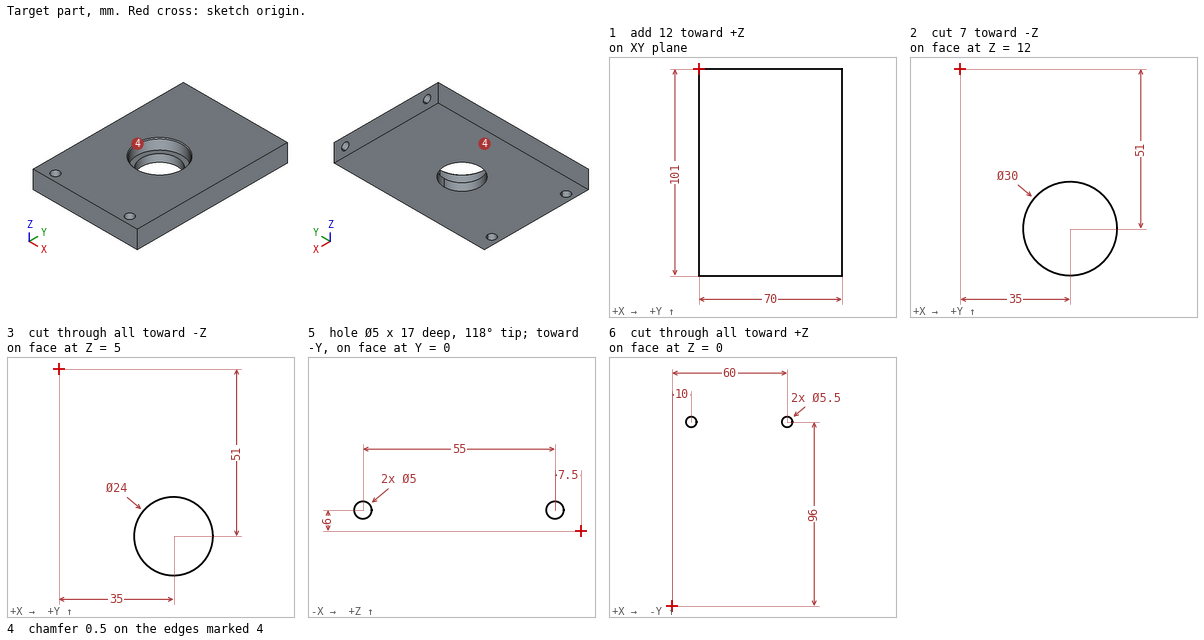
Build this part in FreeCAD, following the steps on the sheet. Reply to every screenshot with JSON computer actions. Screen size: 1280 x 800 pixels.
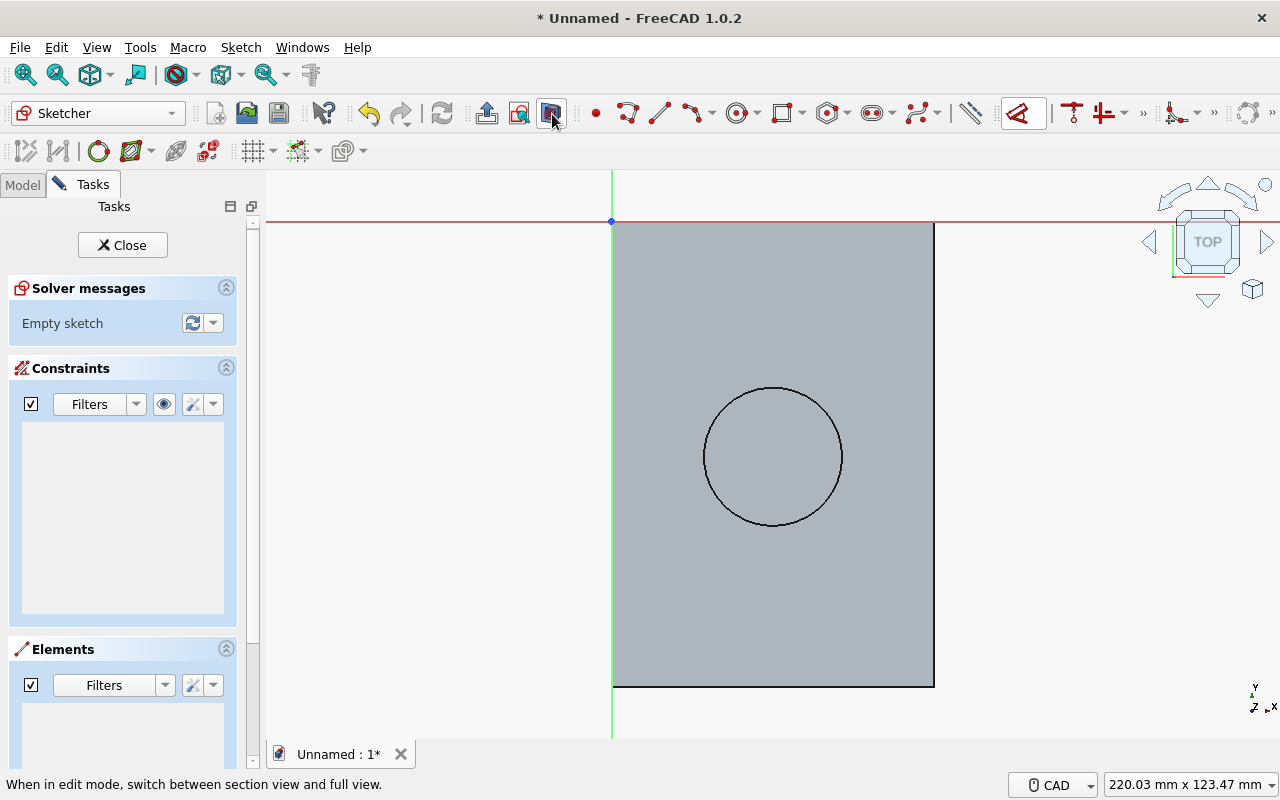
{"action": "scroll", "coordinate": [803, 458], "scroll_direction": "up", "scroll_amount": 6}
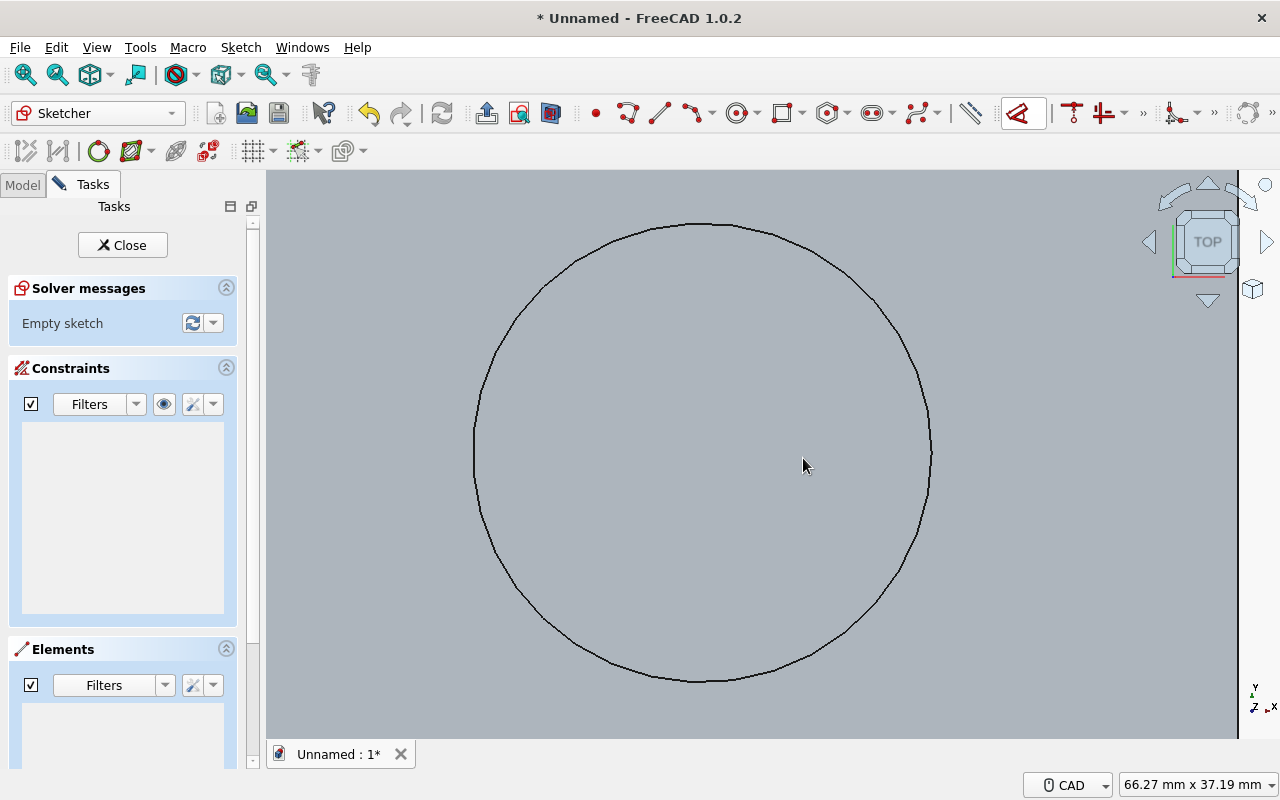
{"action": "left_click", "coordinate": [738, 114]}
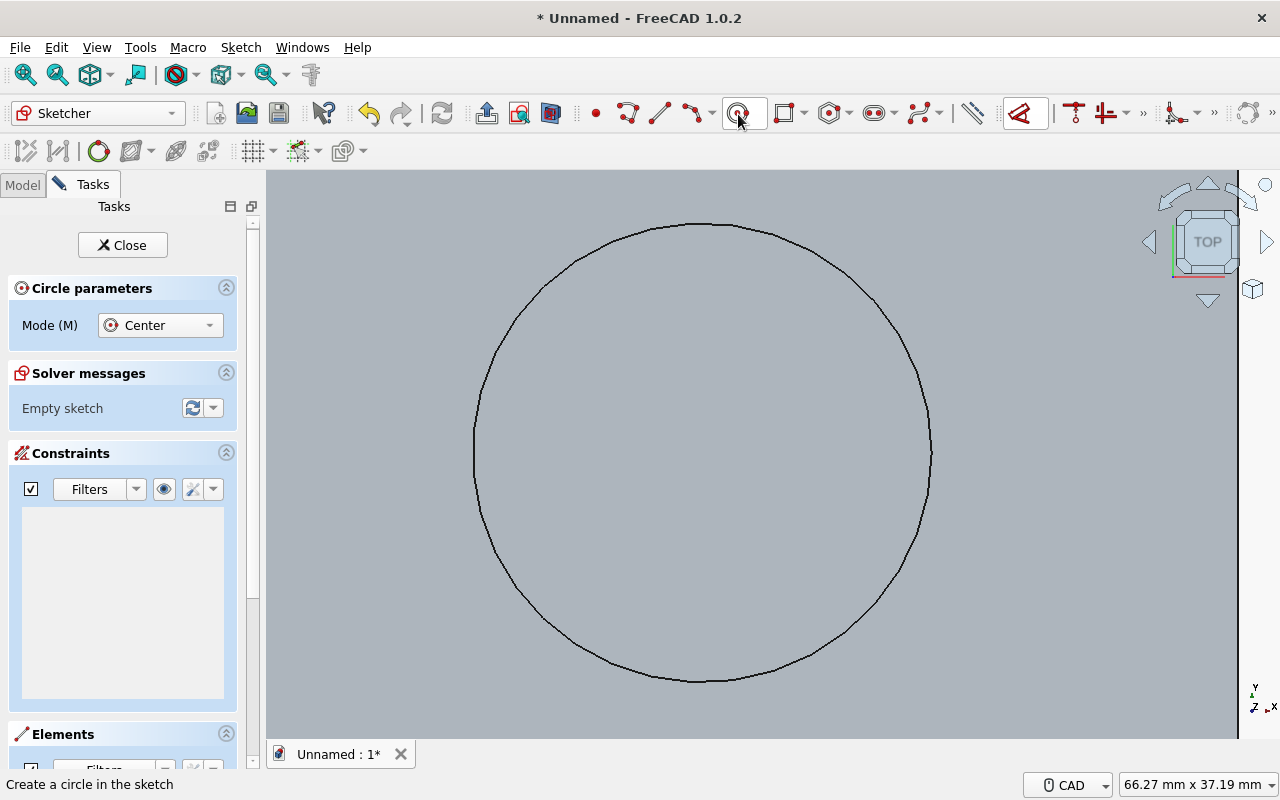
{"action": "left_click", "coordinate": [702, 453]}
{"action": "left_click", "coordinate": [832, 323]}
{"action": "key", "text": "Escape"}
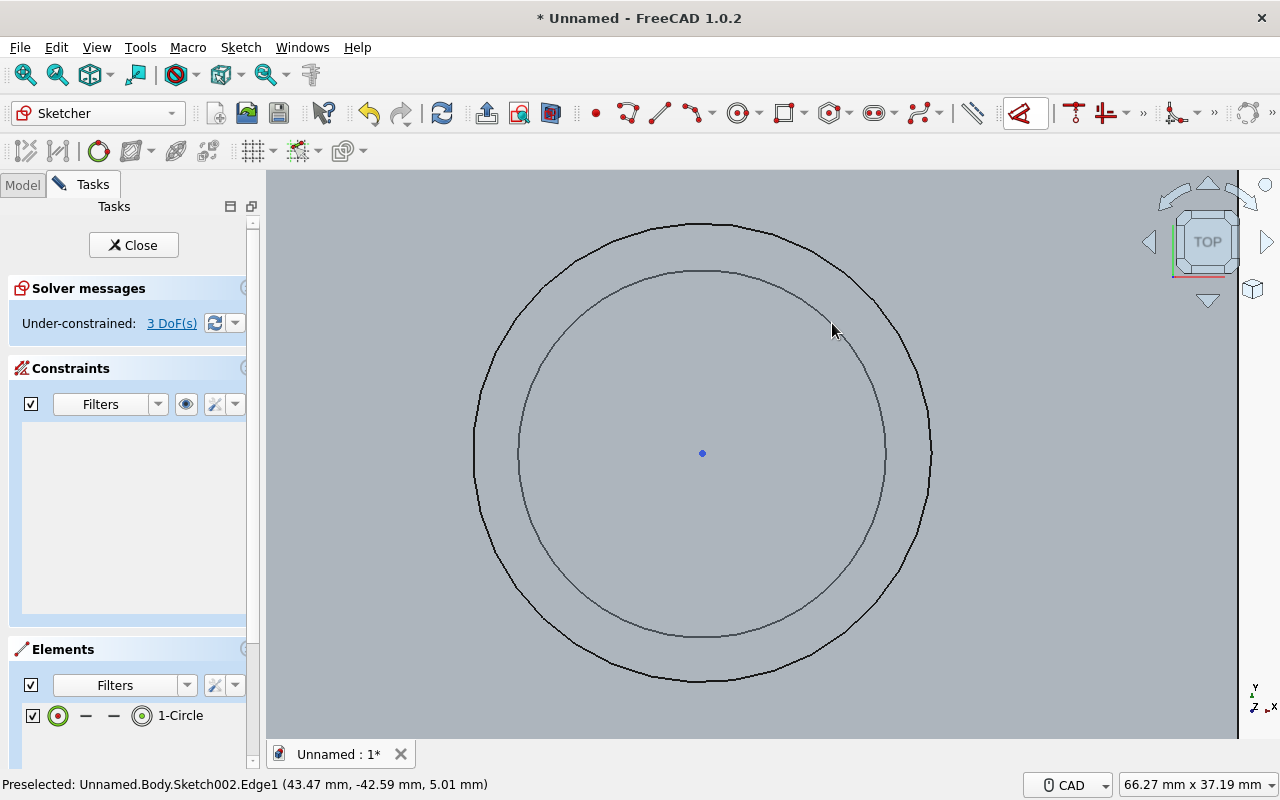
{"action": "left_click", "coordinate": [832, 324]}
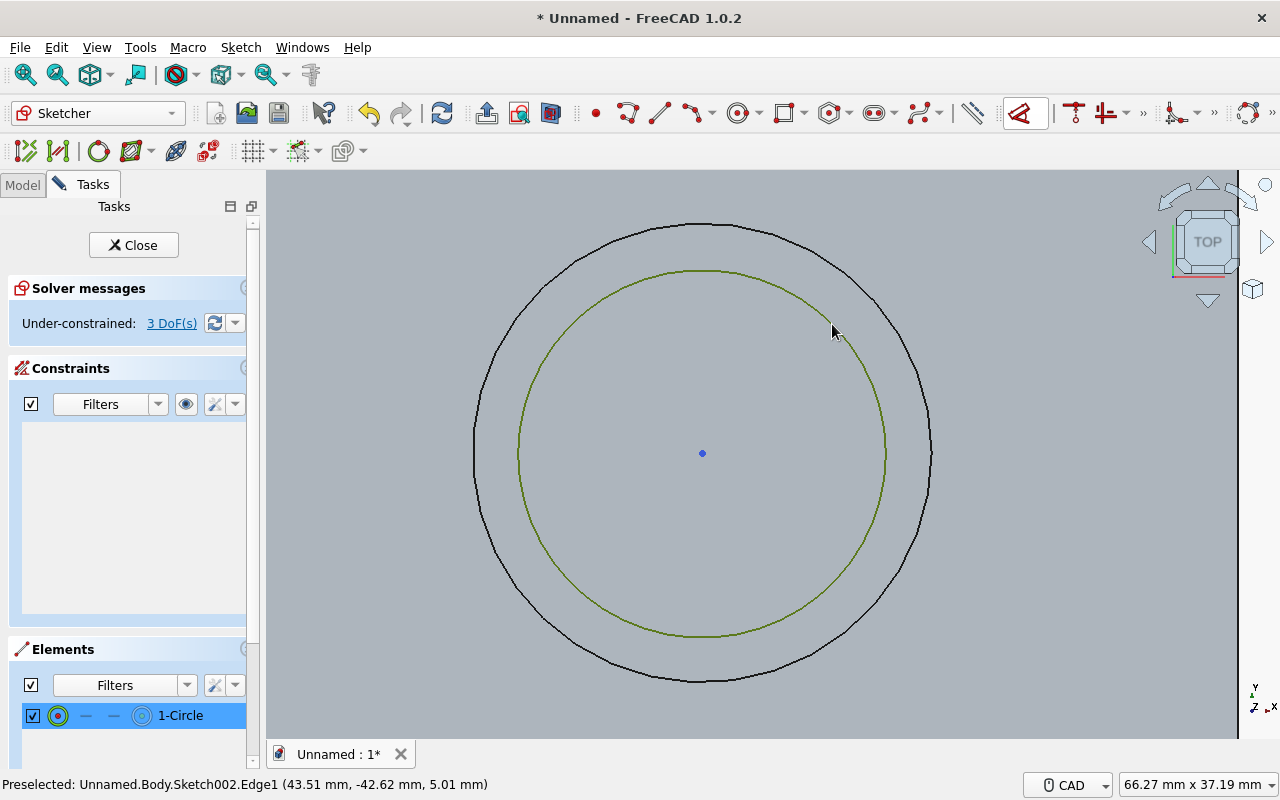
{"action": "key", "text": "k o"}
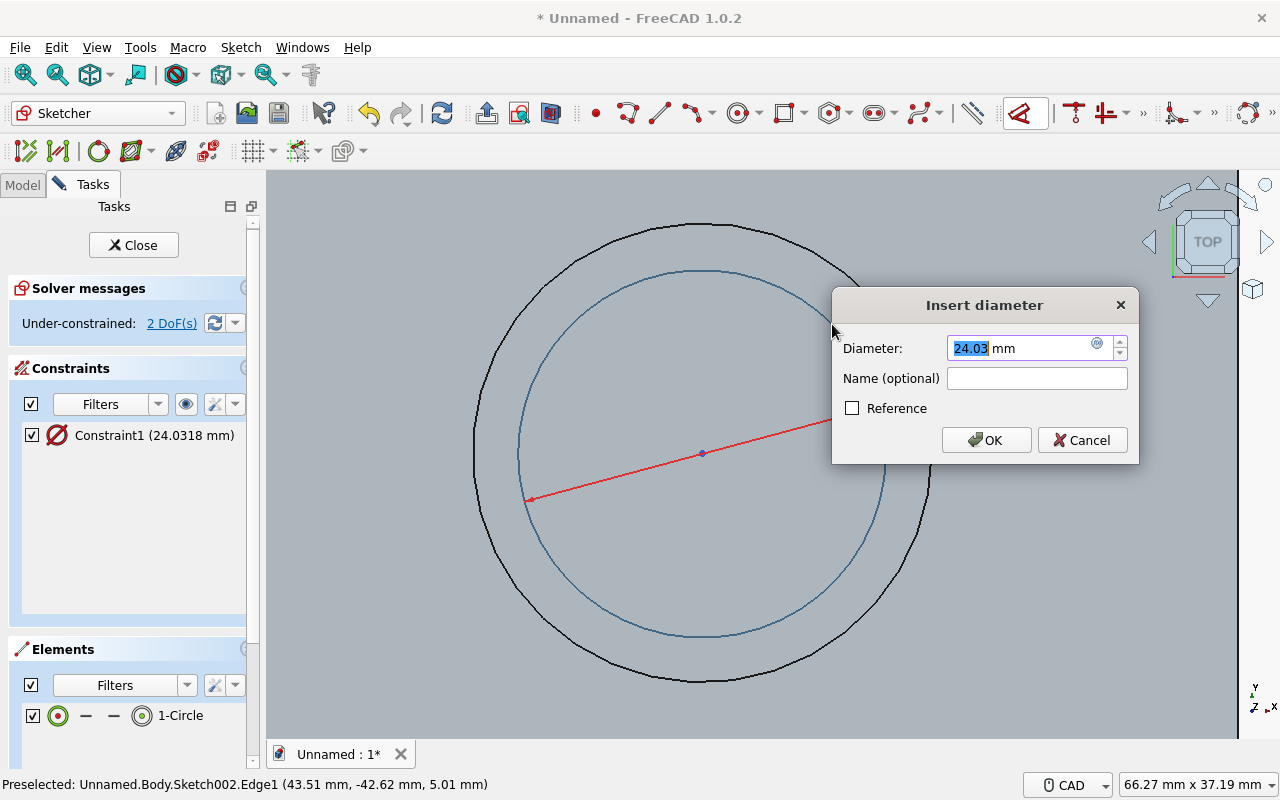
{"action": "type", "text": "24"}
{"action": "key", "text": "Return"}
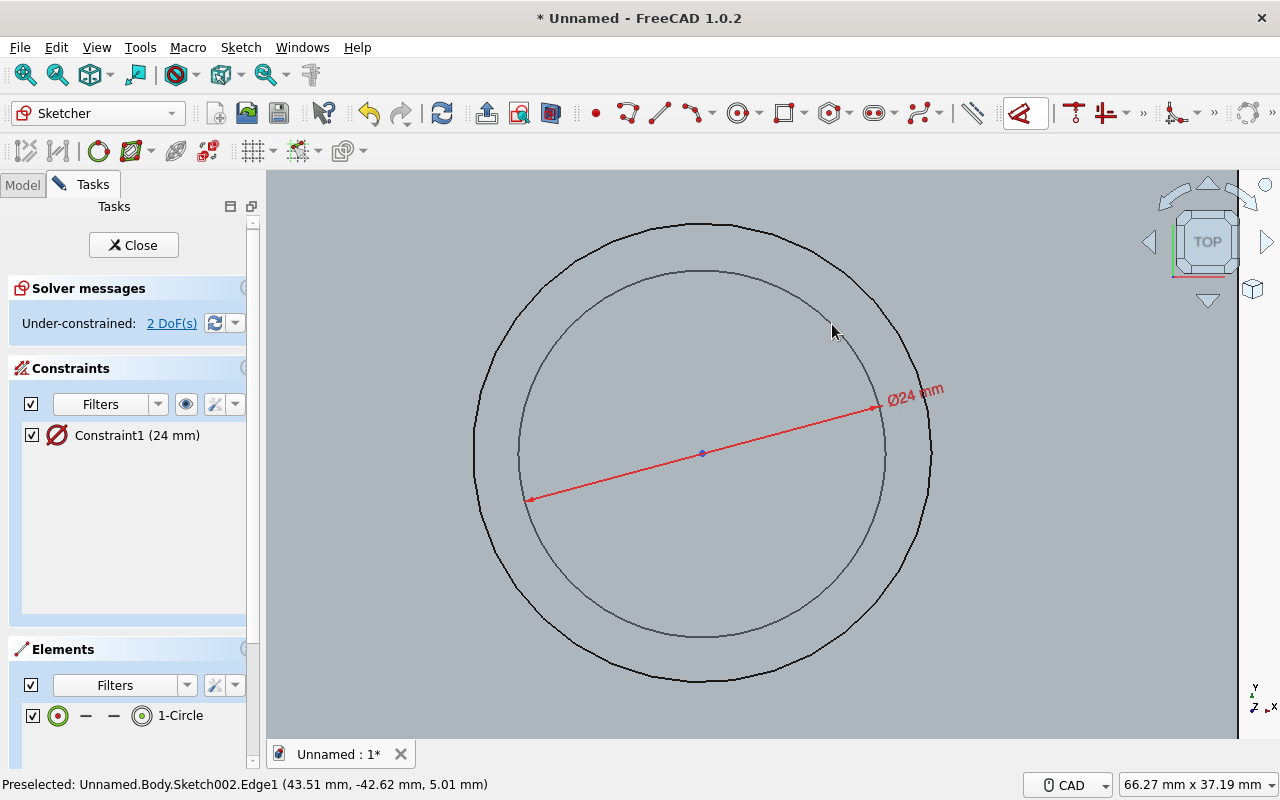
{"action": "left_click", "coordinate": [702, 454]}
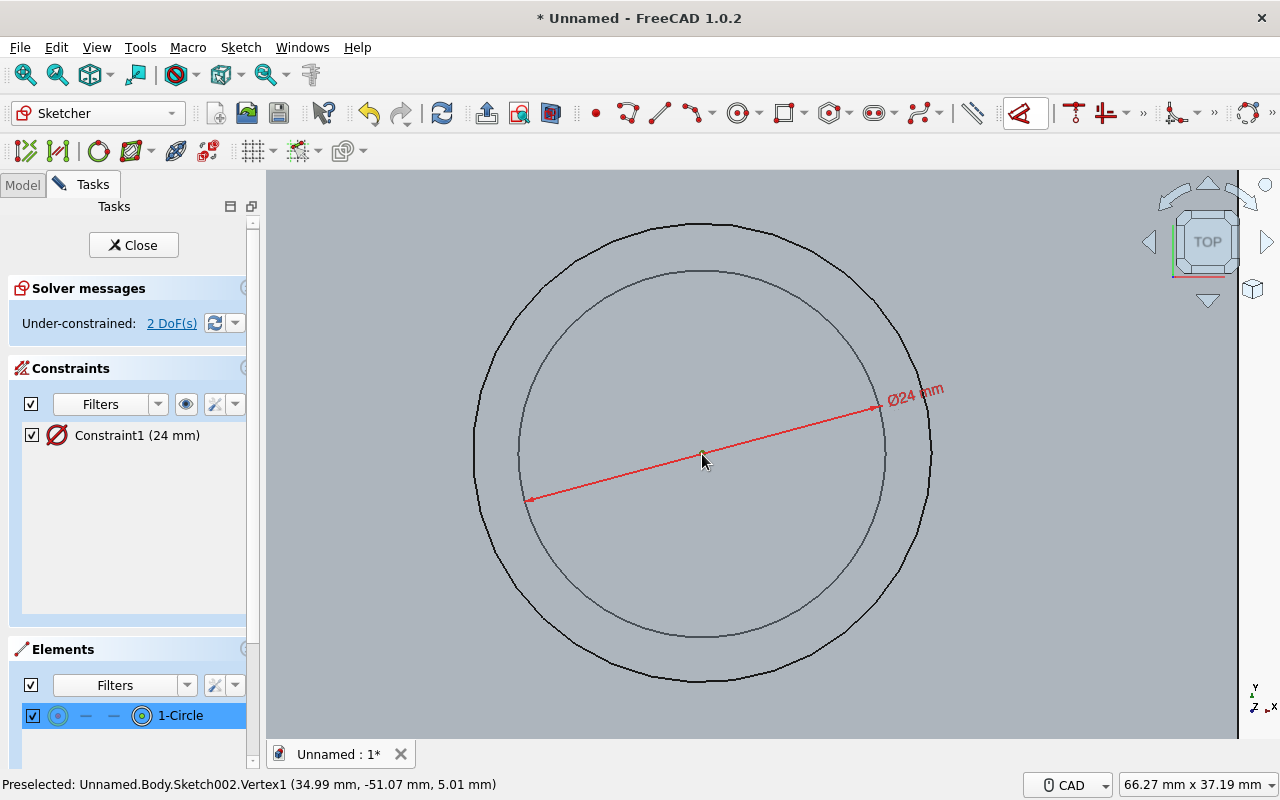
{"action": "left_click", "coordinate": [1042, 114]}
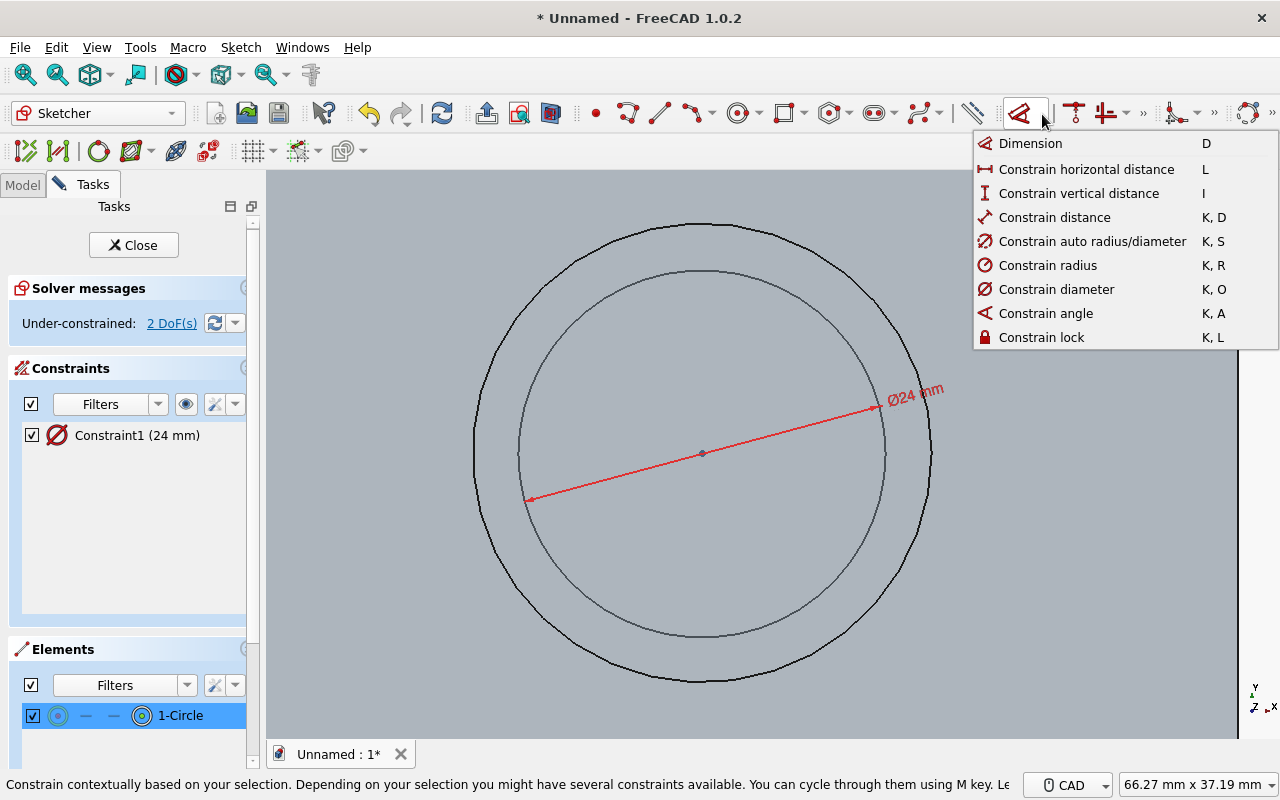
{"action": "left_click", "coordinate": [1126, 169]}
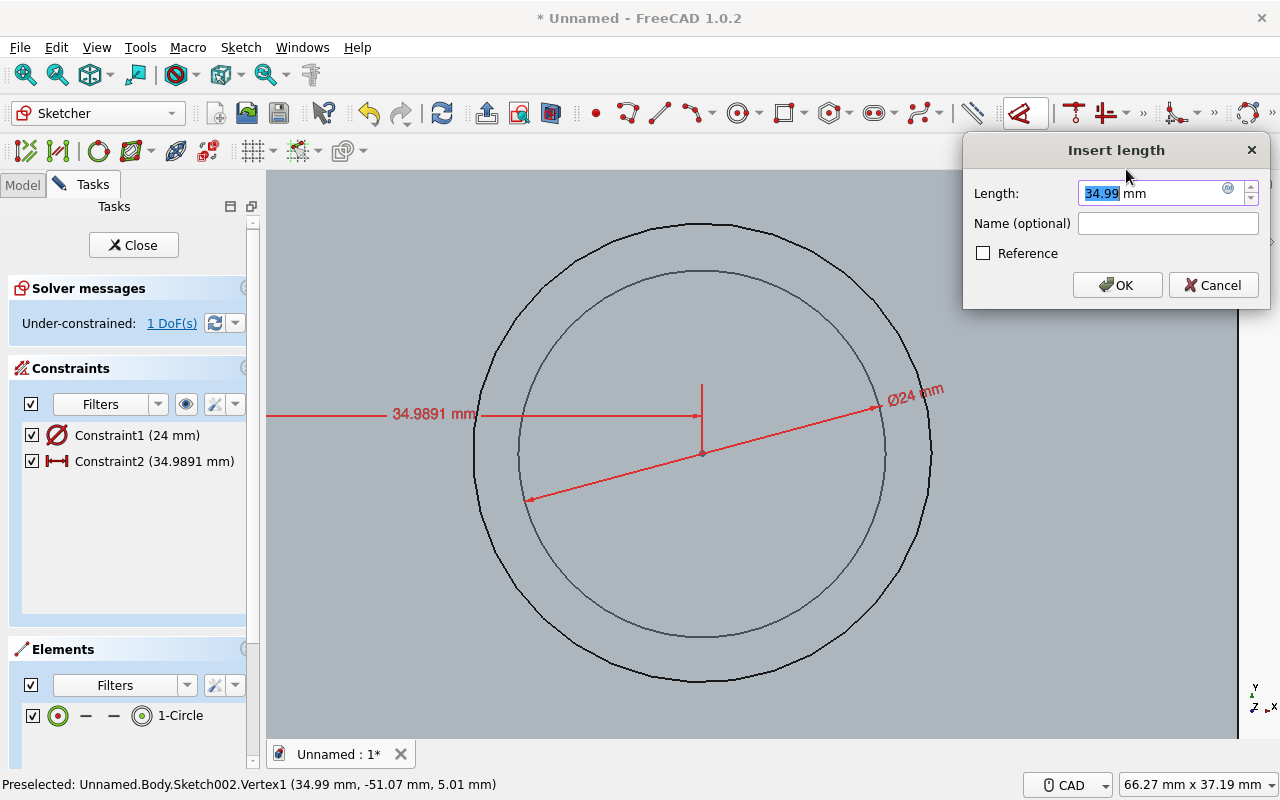
{"action": "type", "text": "35"}
{"action": "key", "text": "Return"}